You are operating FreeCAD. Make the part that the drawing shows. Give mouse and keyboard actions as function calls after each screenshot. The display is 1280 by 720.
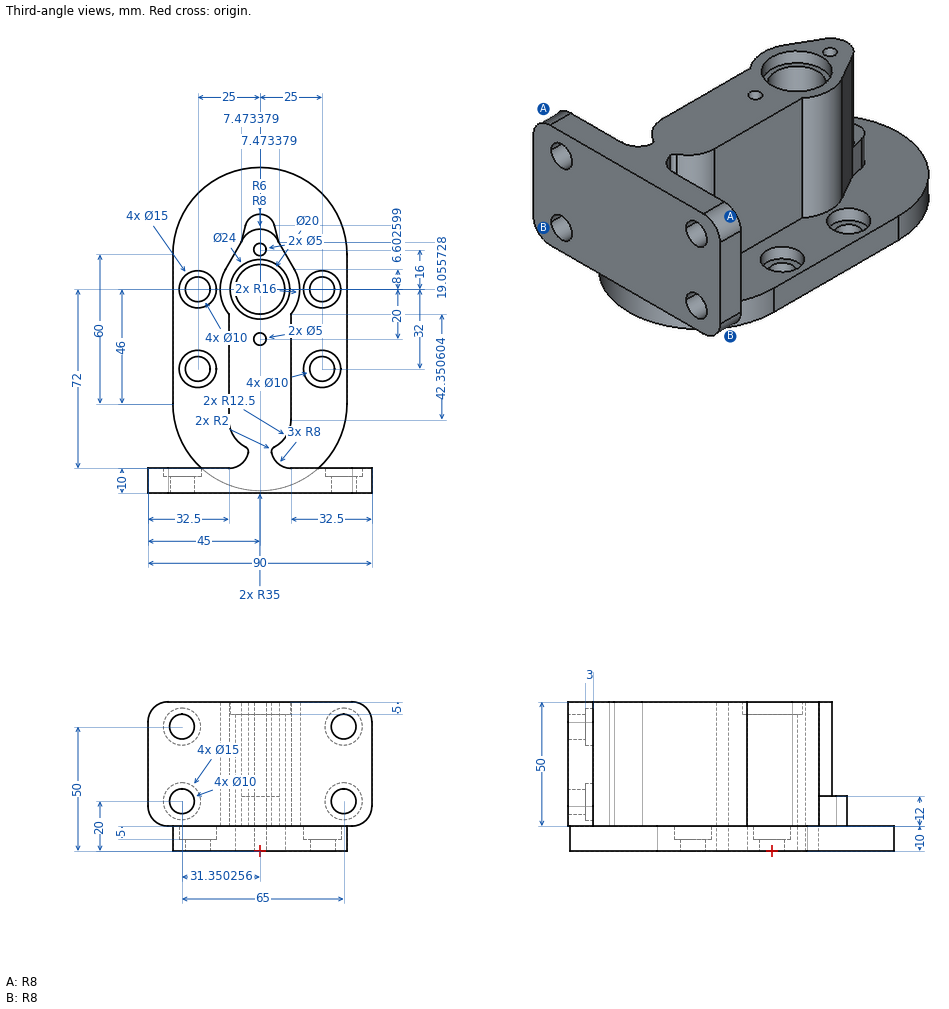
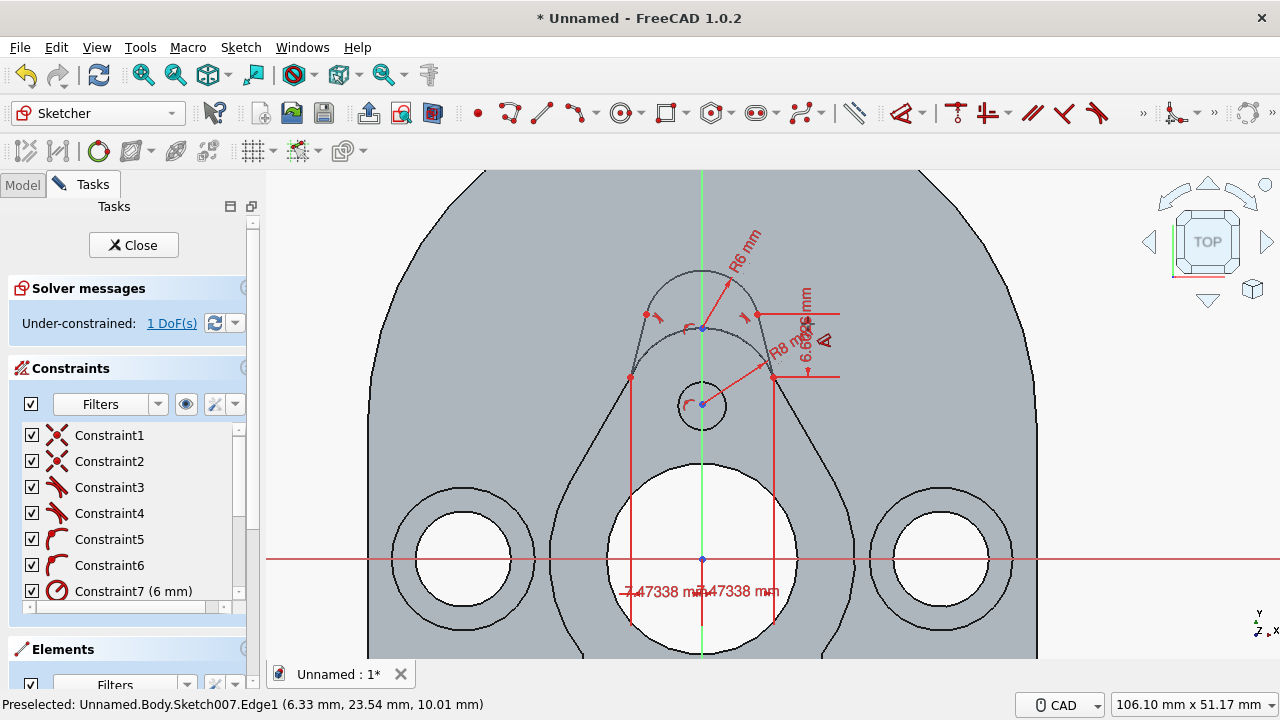
click(774, 377)
click(808, 468)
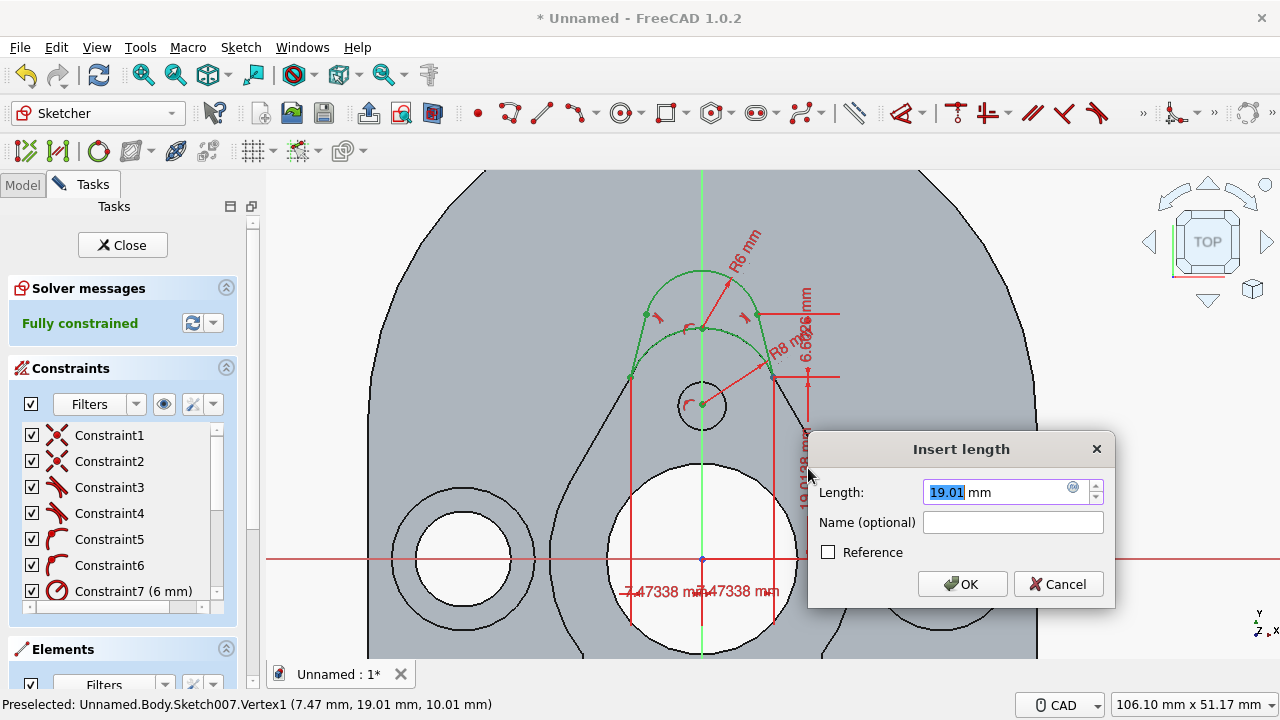
text(19.055728)
key(Return)
key(Escape)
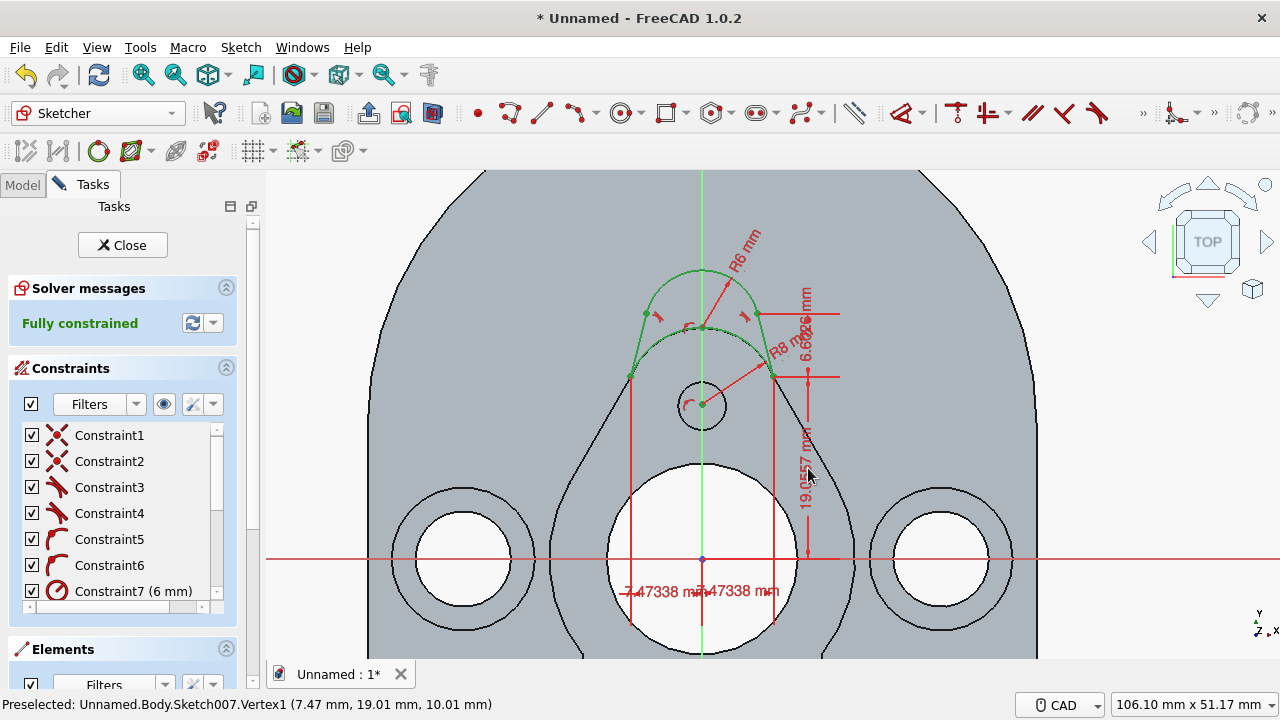
click(123, 245)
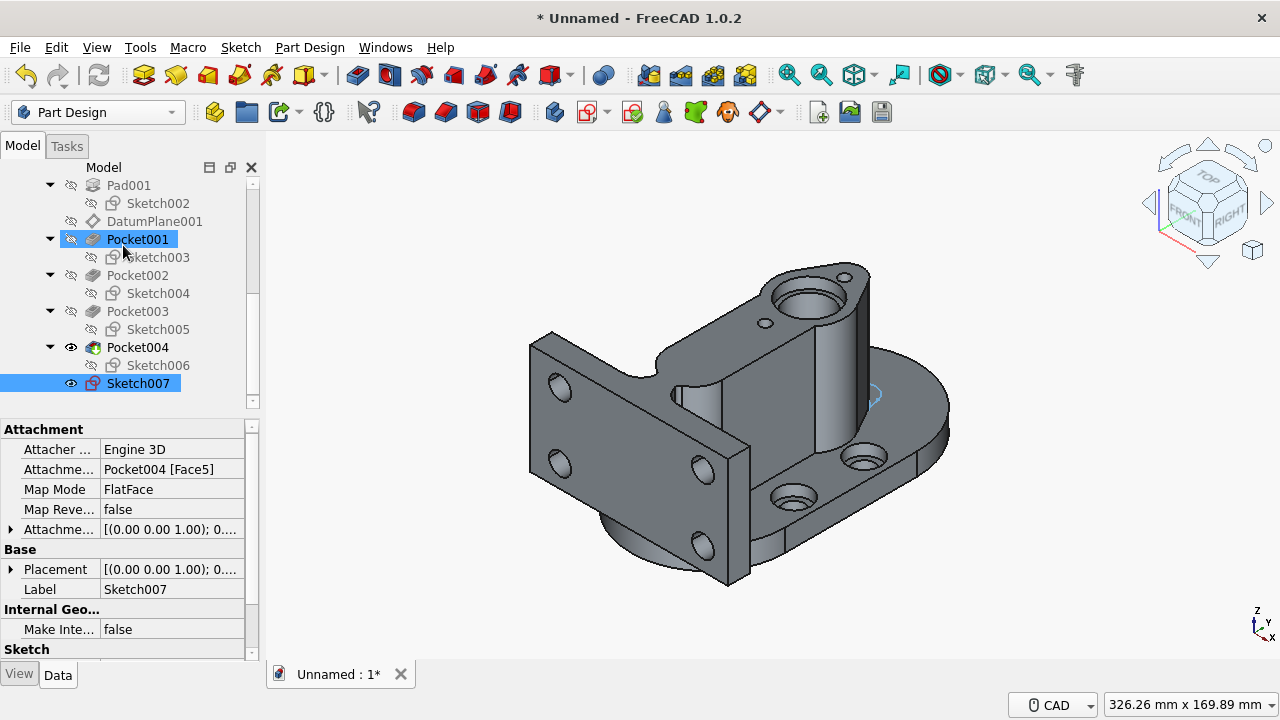
click(144, 76)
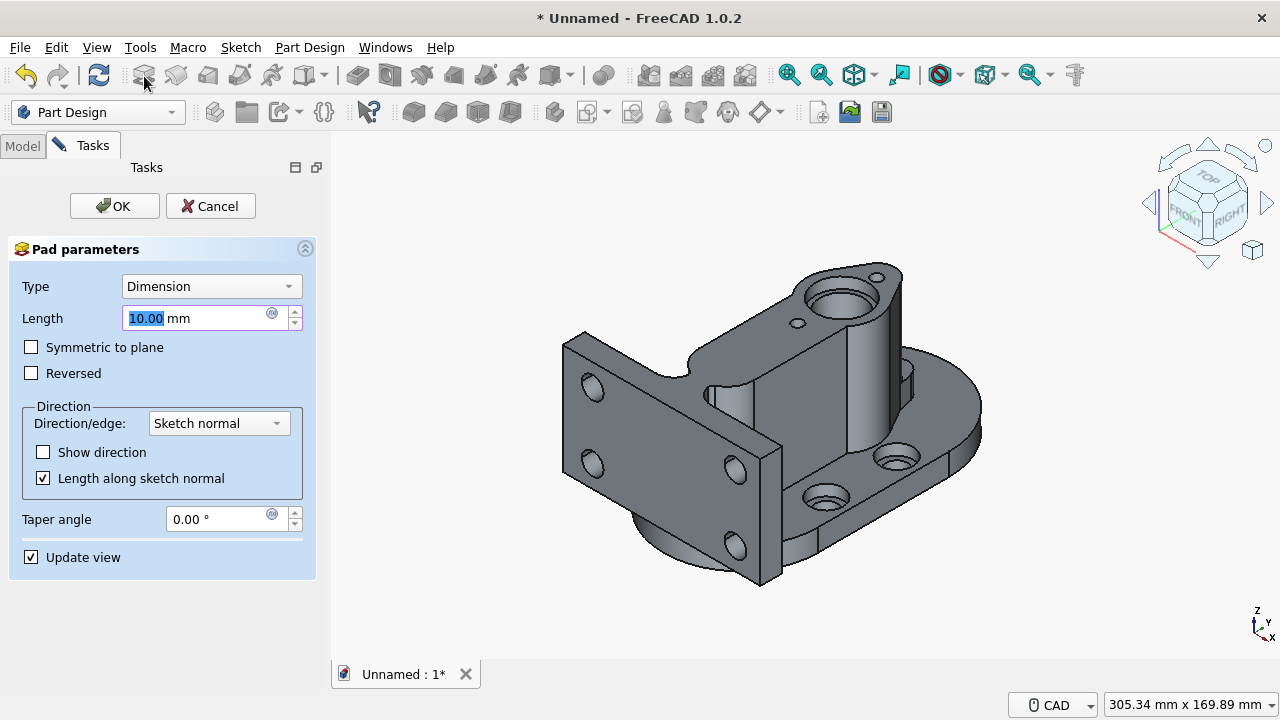
text(12)
key(Tab)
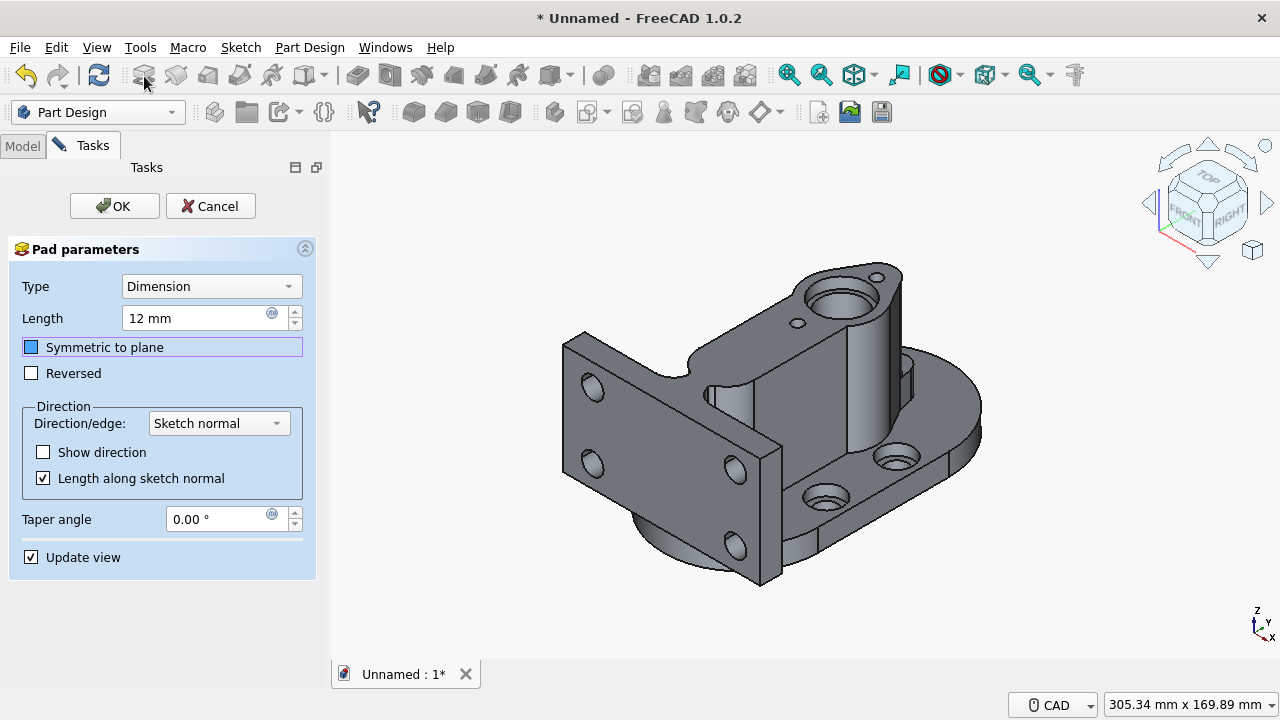
click(115, 206)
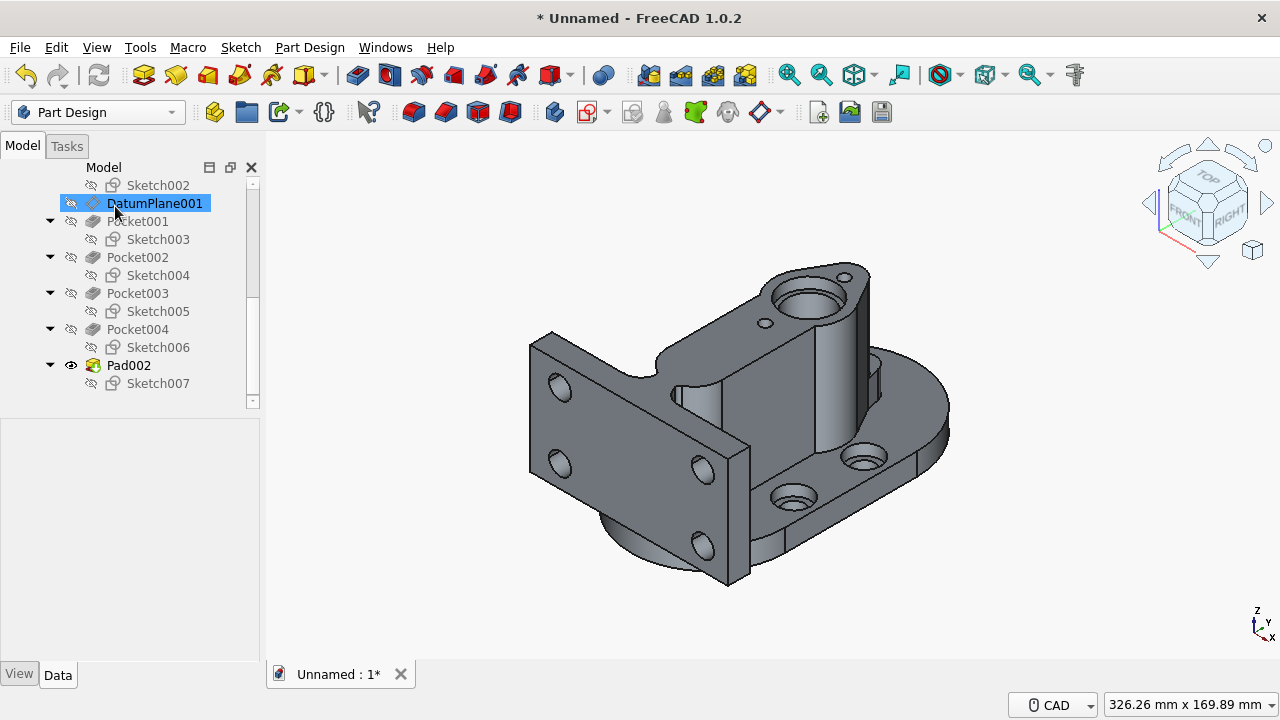
click(739, 452)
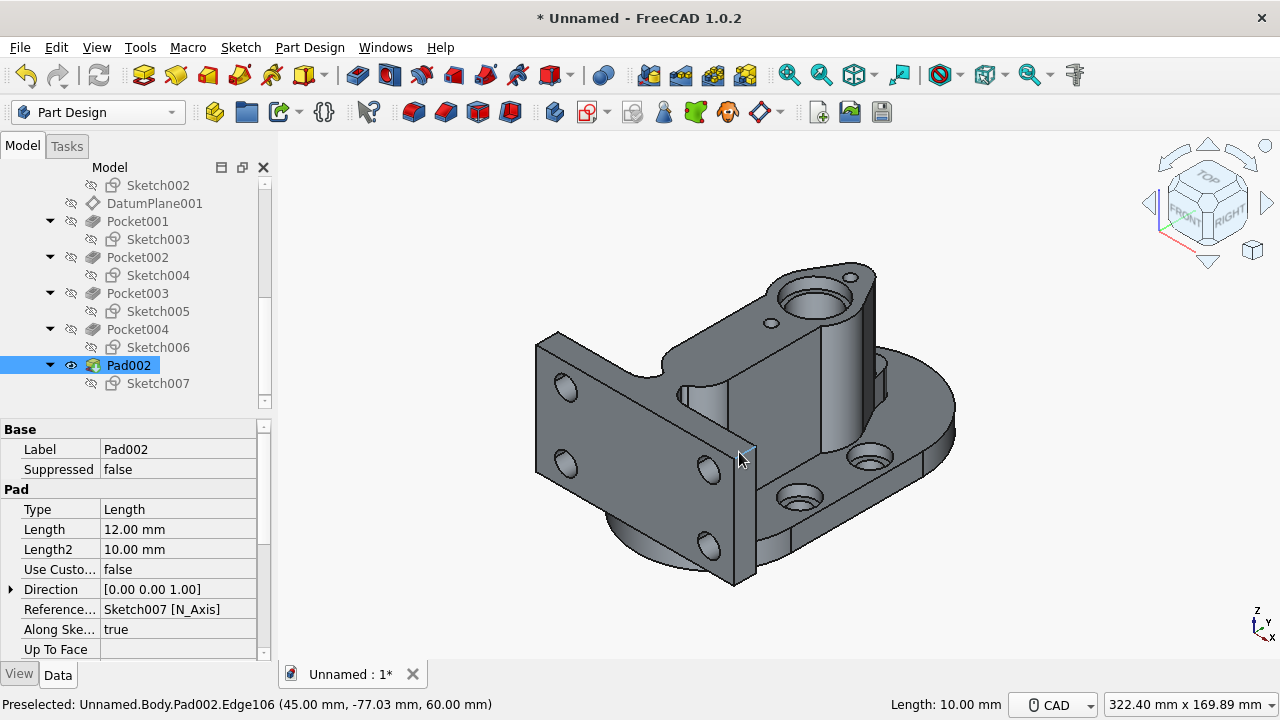
key(2)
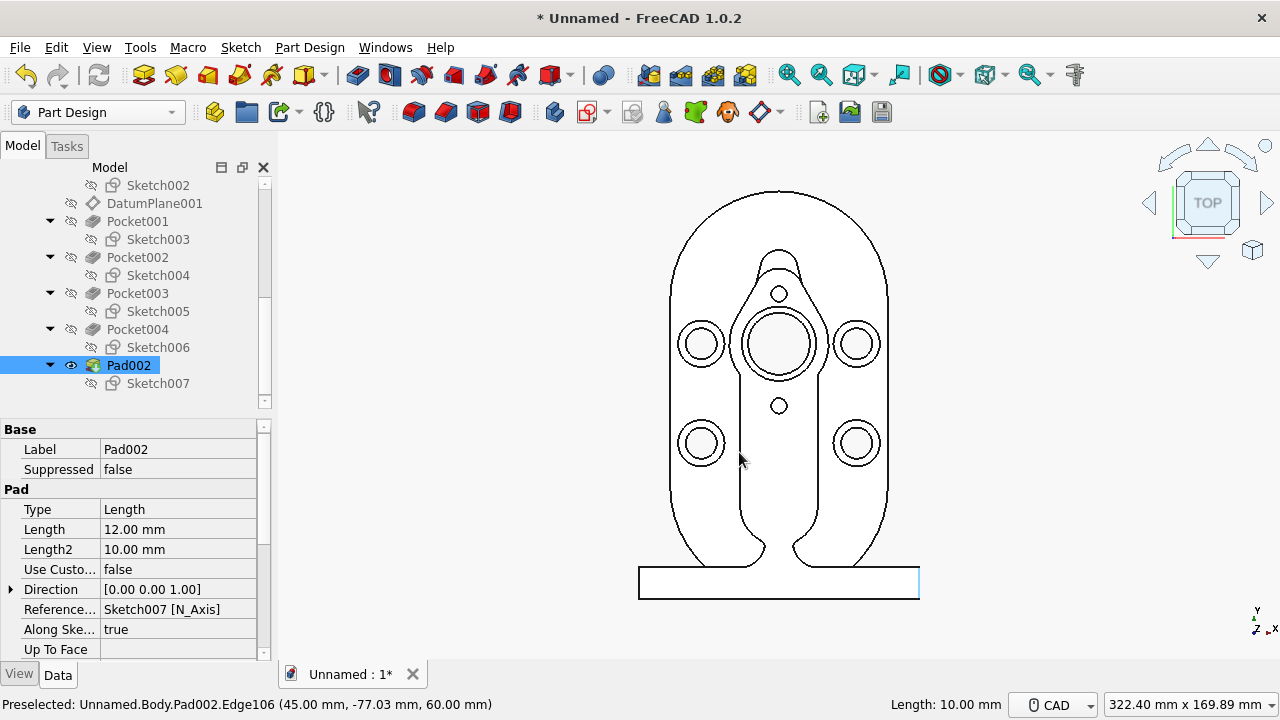
click(639, 582, ctrl)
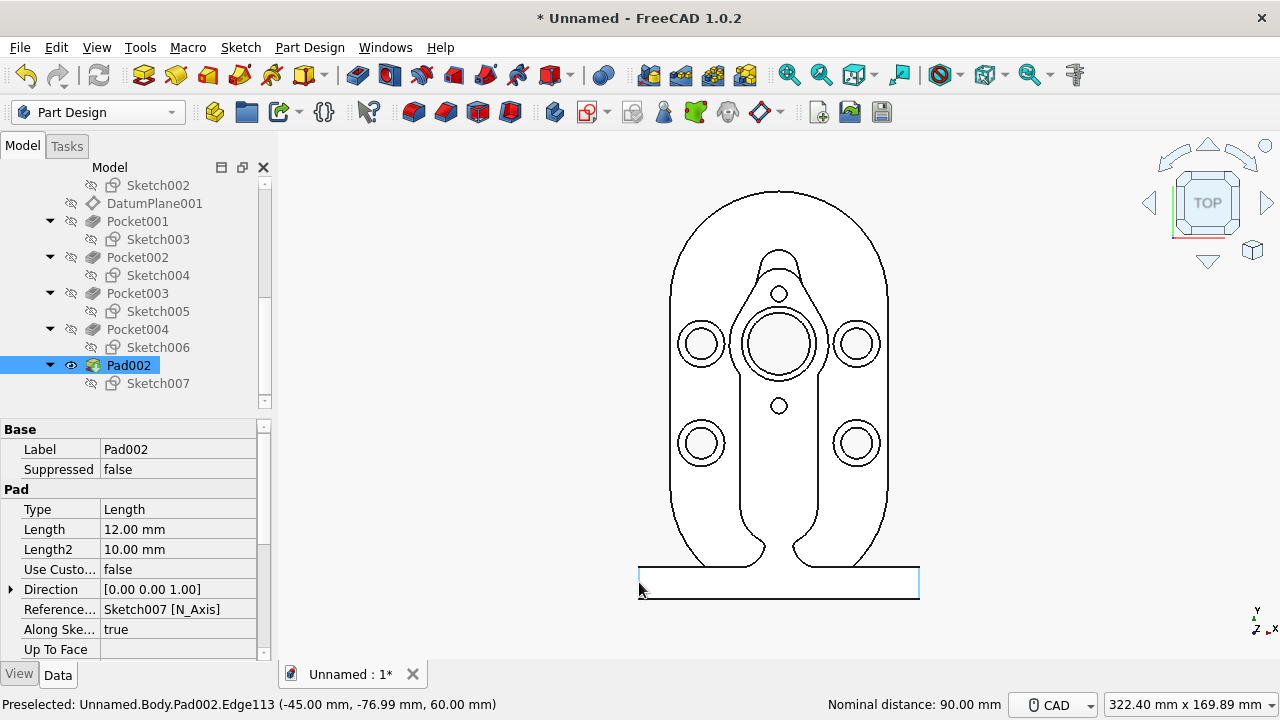
click(414, 112)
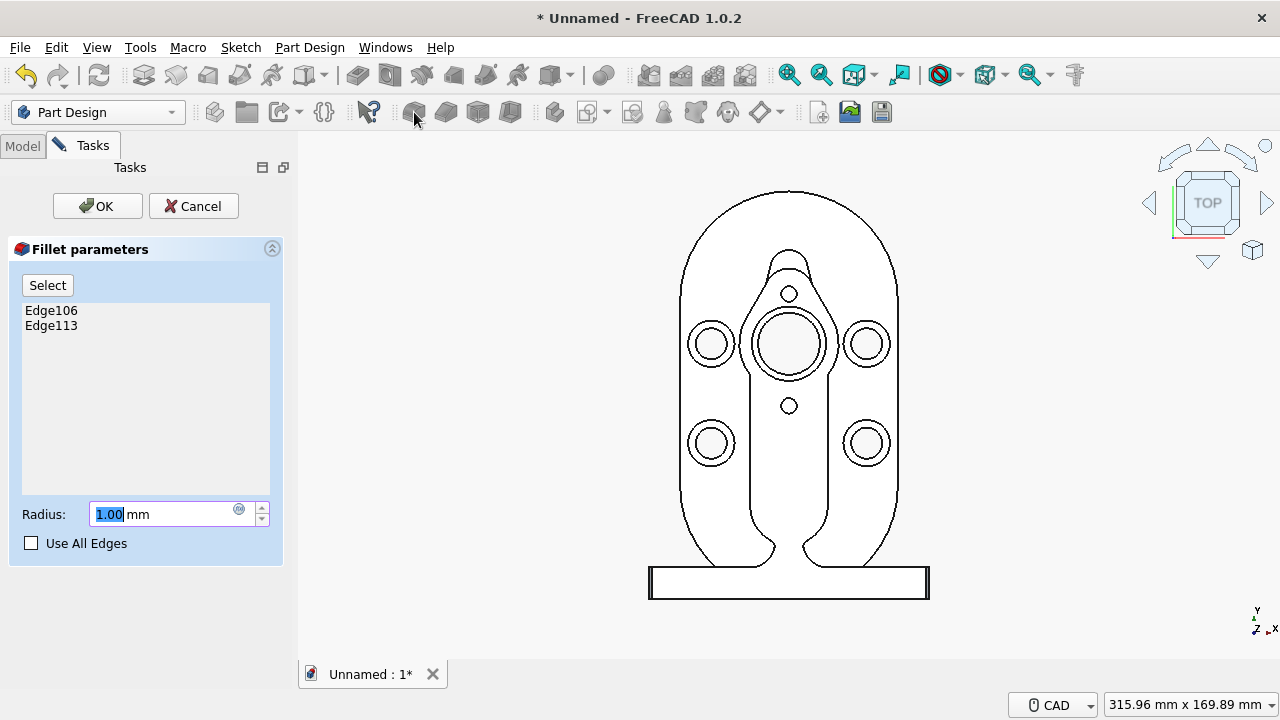
text(8)
key(Tab)